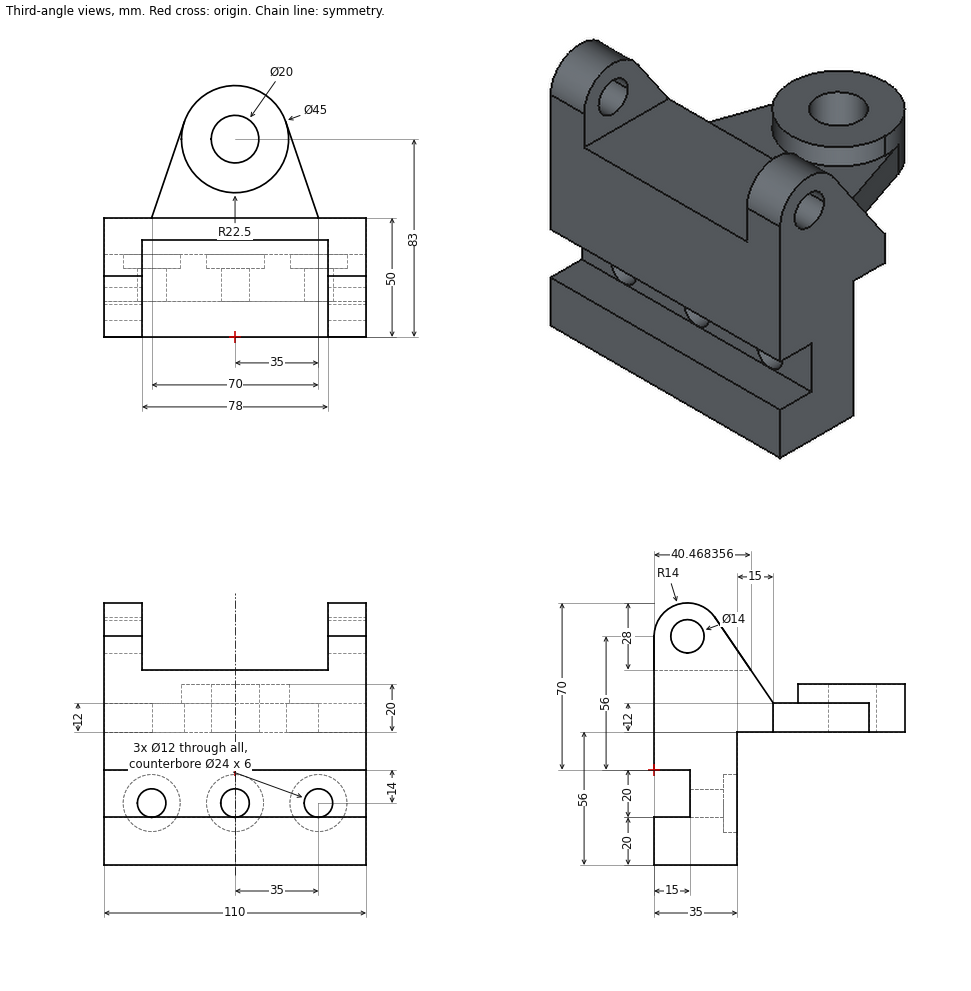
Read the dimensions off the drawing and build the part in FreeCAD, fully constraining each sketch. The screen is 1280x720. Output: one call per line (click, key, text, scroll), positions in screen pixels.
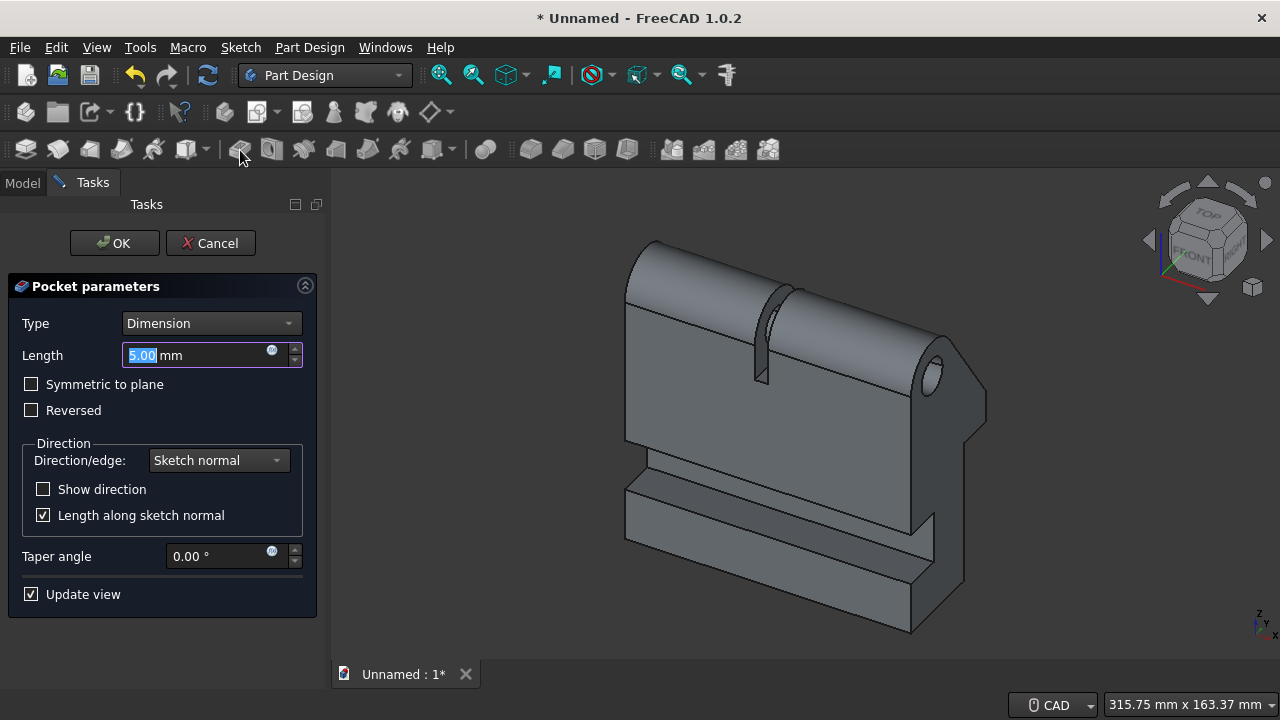
text(78)
key(Tab)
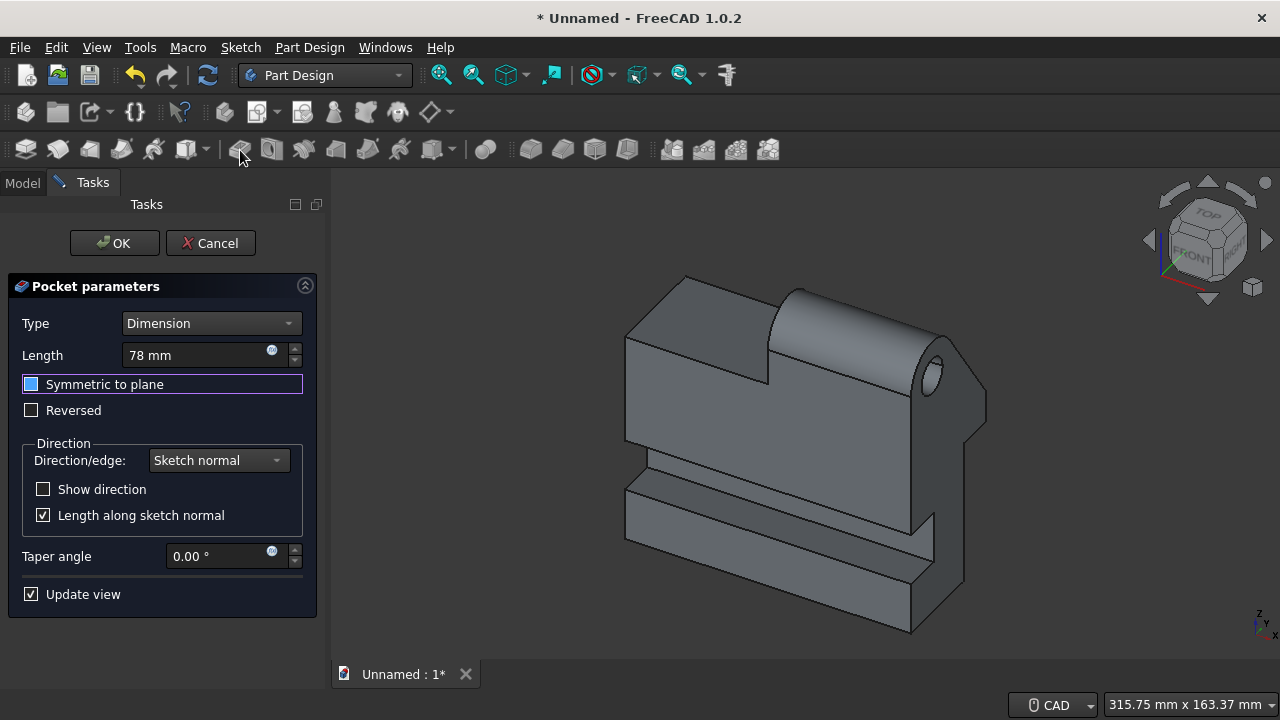
click(30, 384)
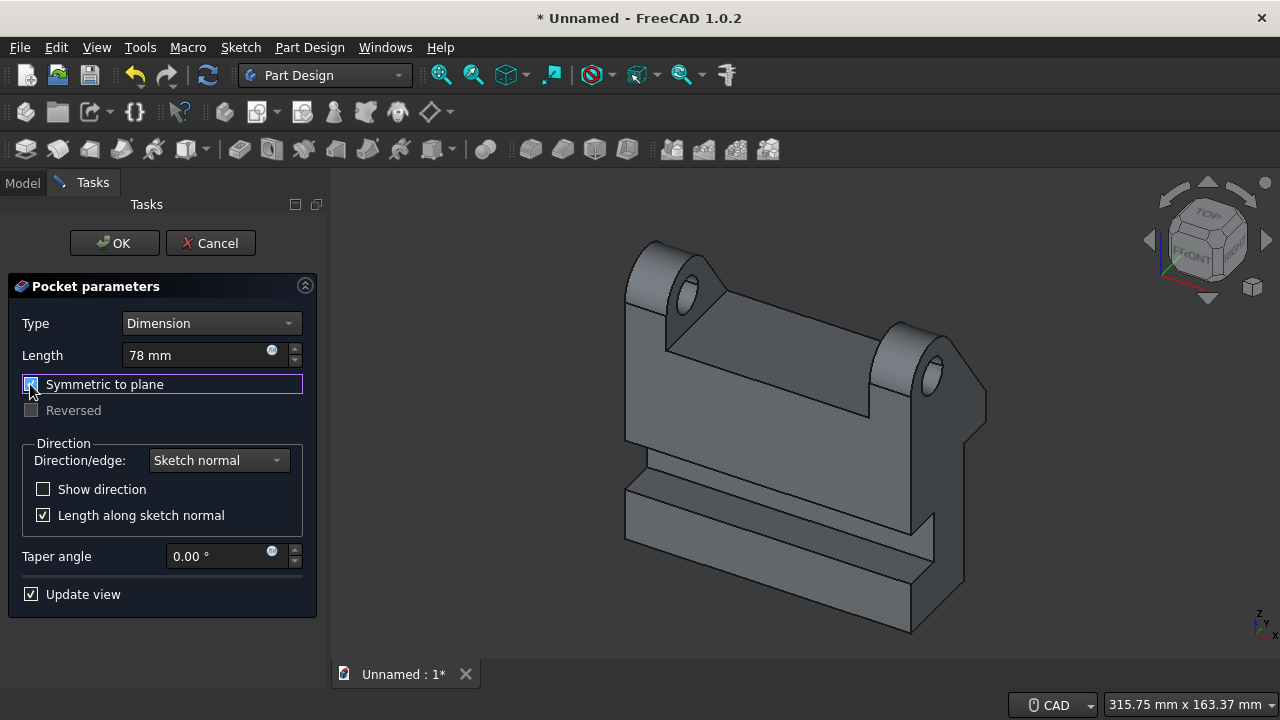
click(115, 243)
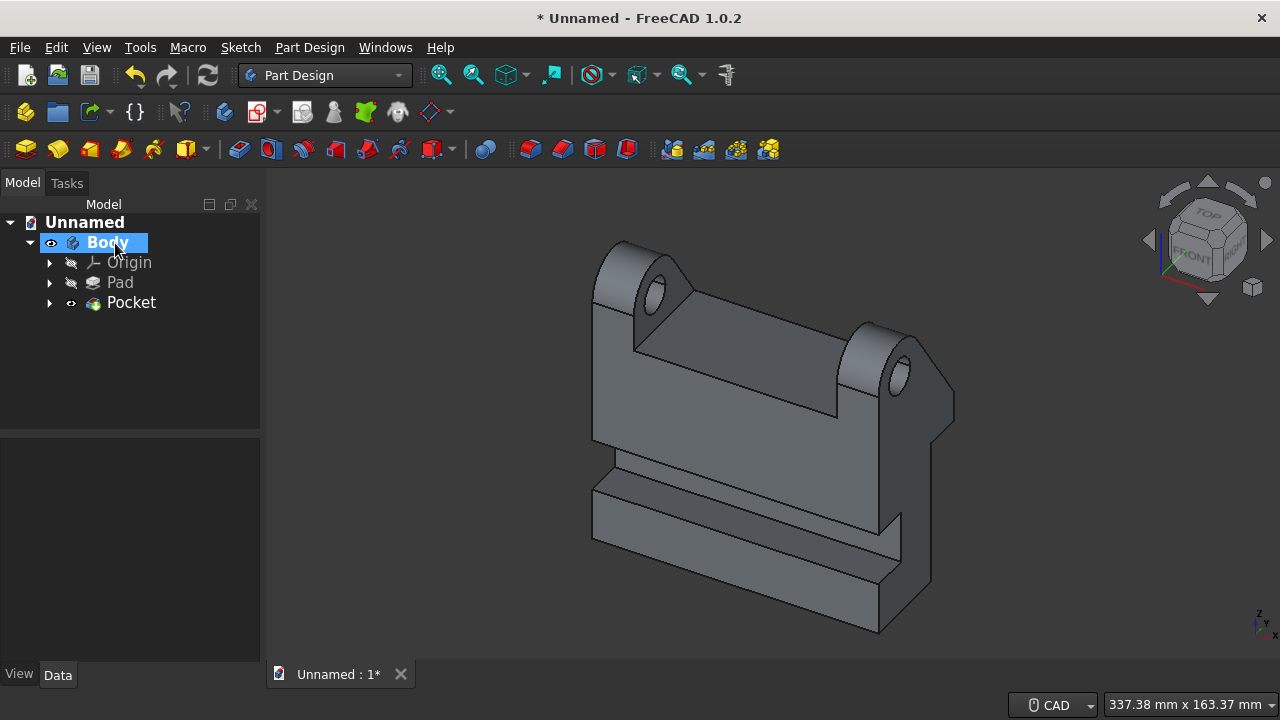
click(226, 112)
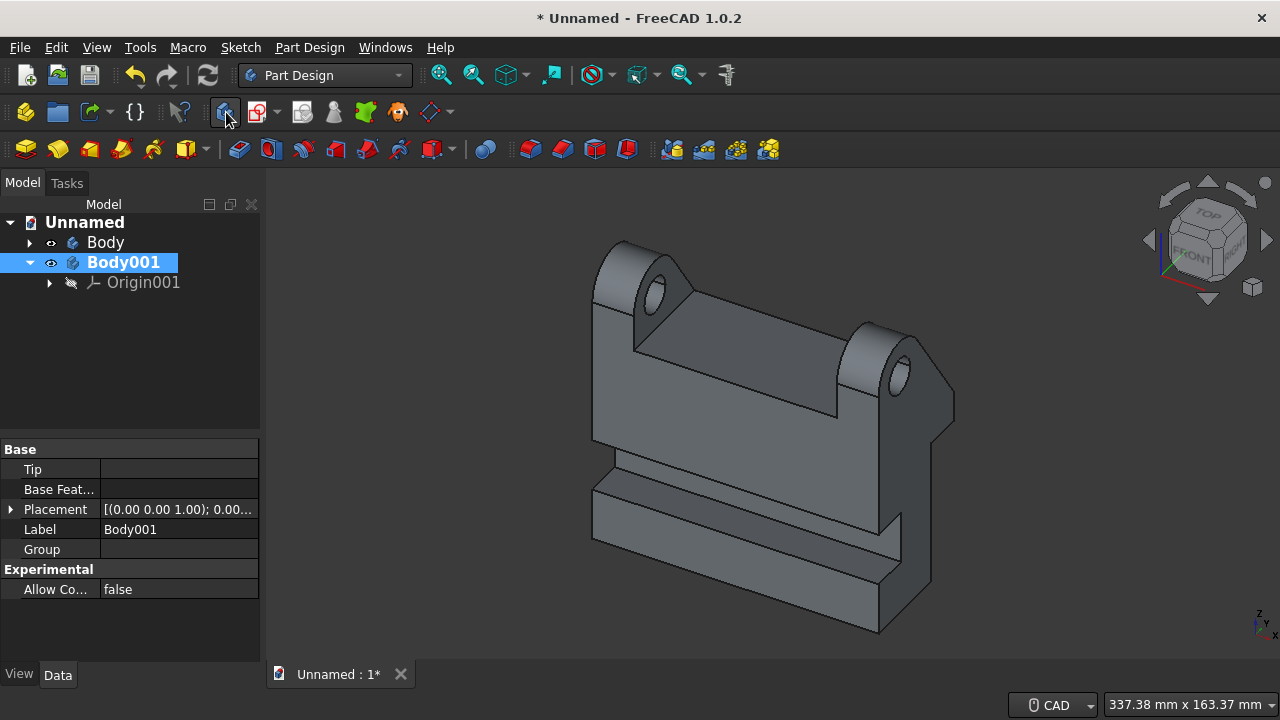
click(50, 283)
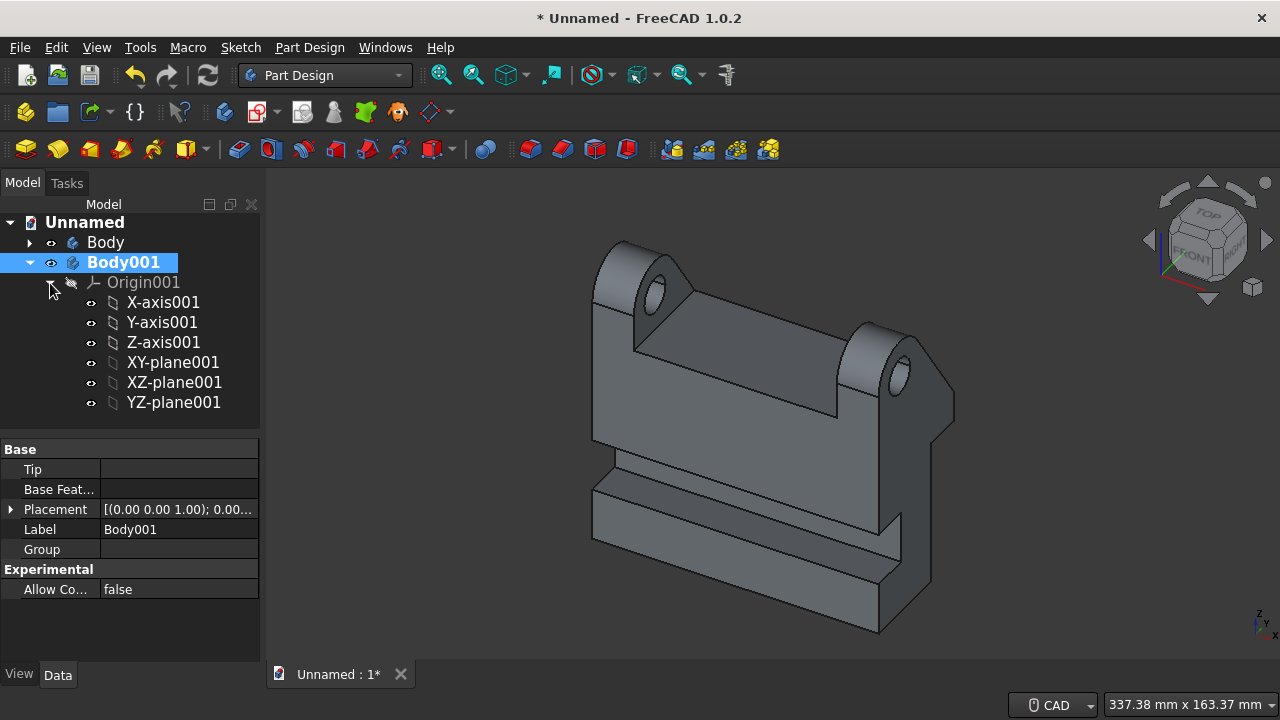
click(136, 363)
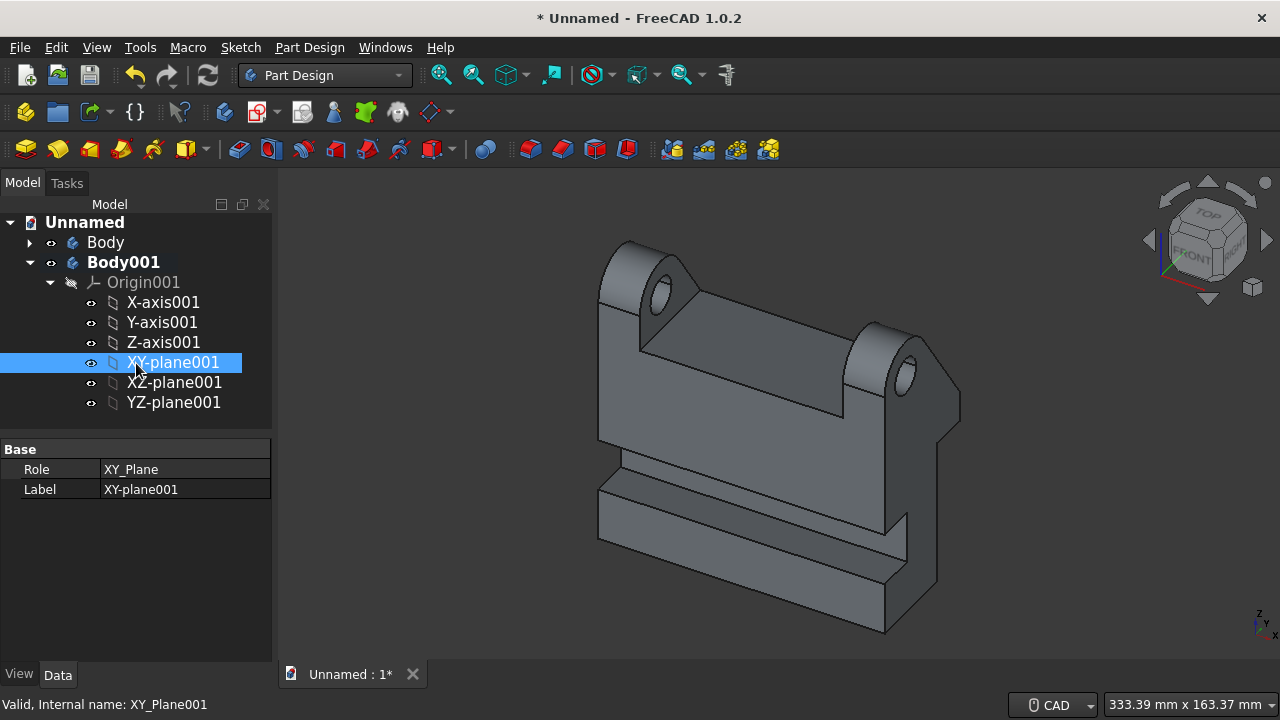
click(430, 112)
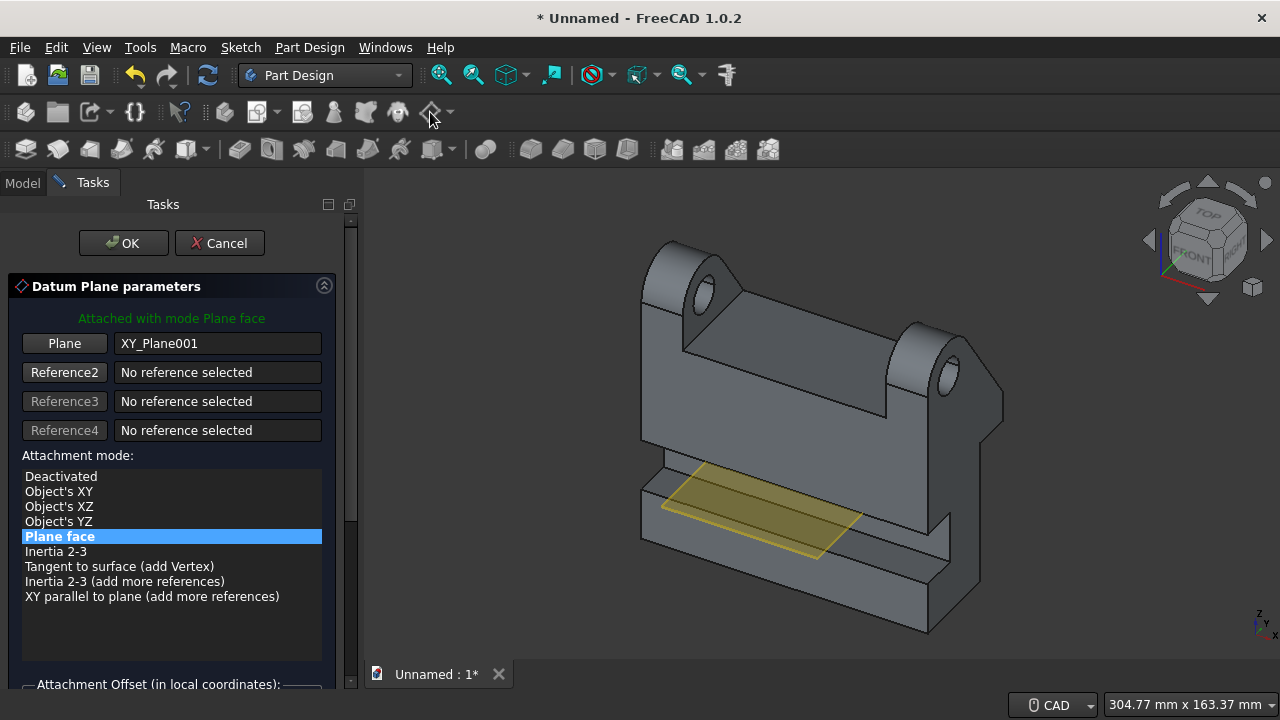
scroll(351, 451, down, 3)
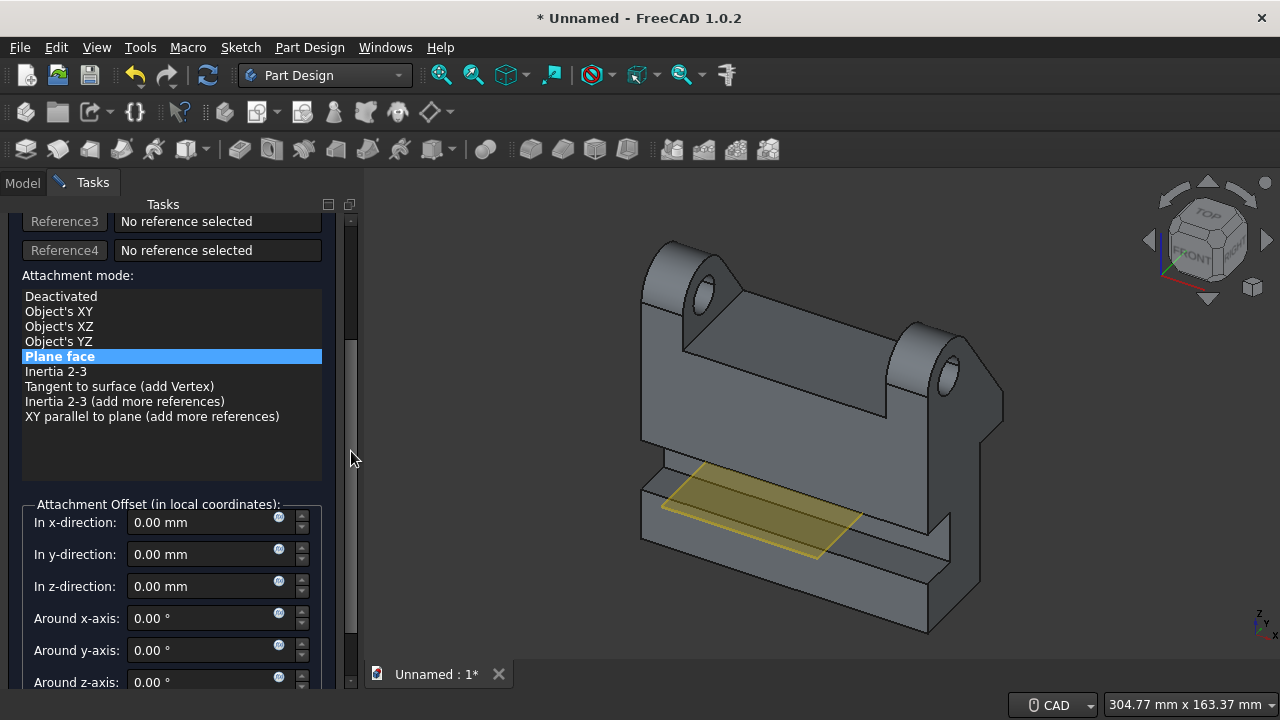
triple_click(210, 586)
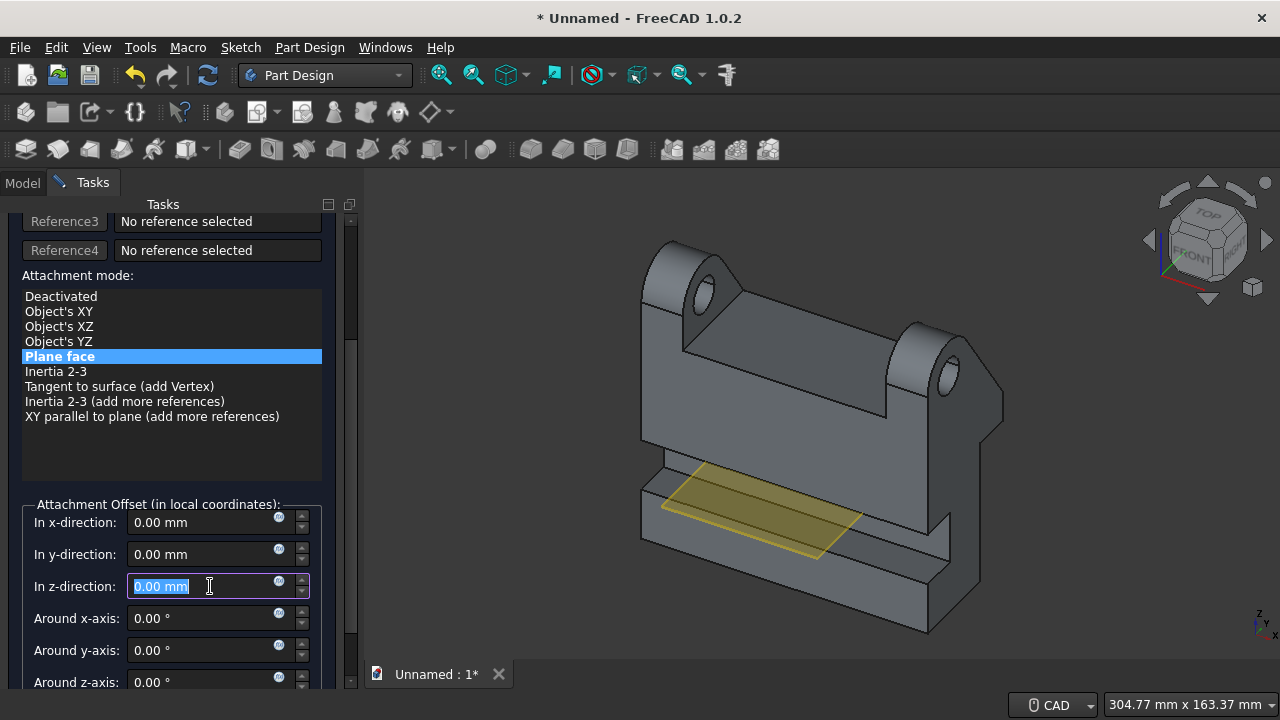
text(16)
key(Tab)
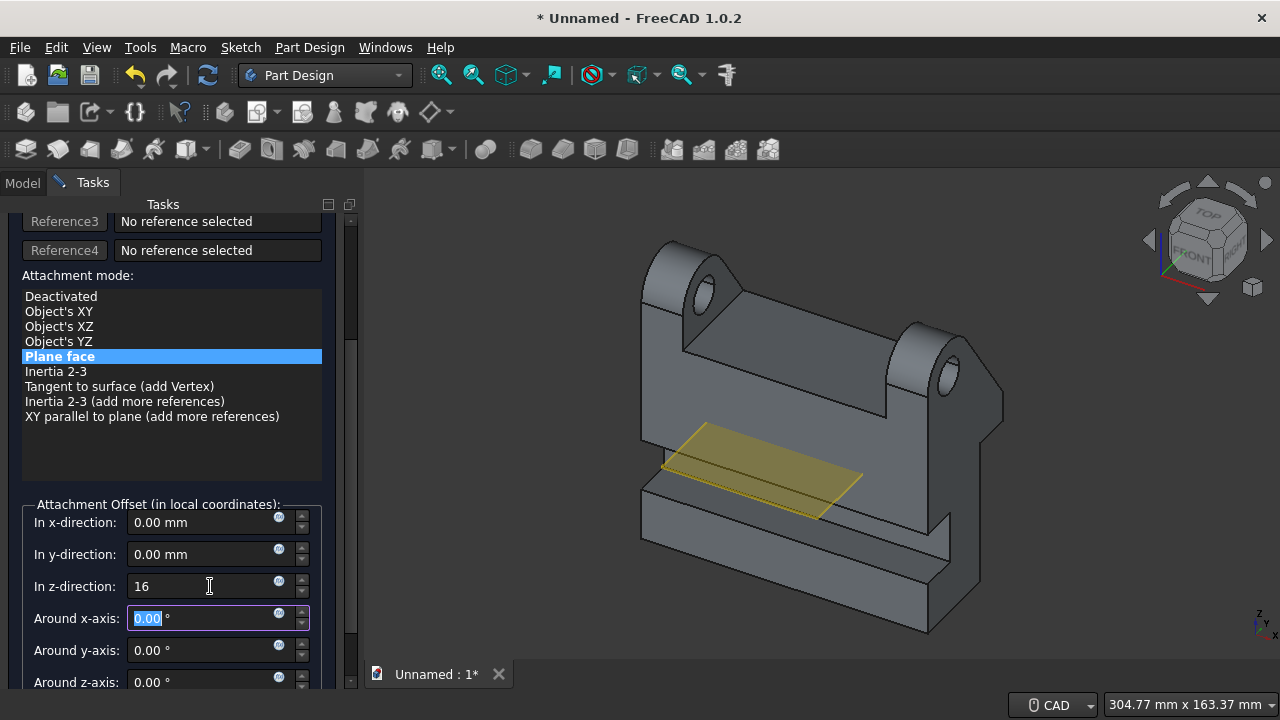
scroll(351, 451, up, 4)